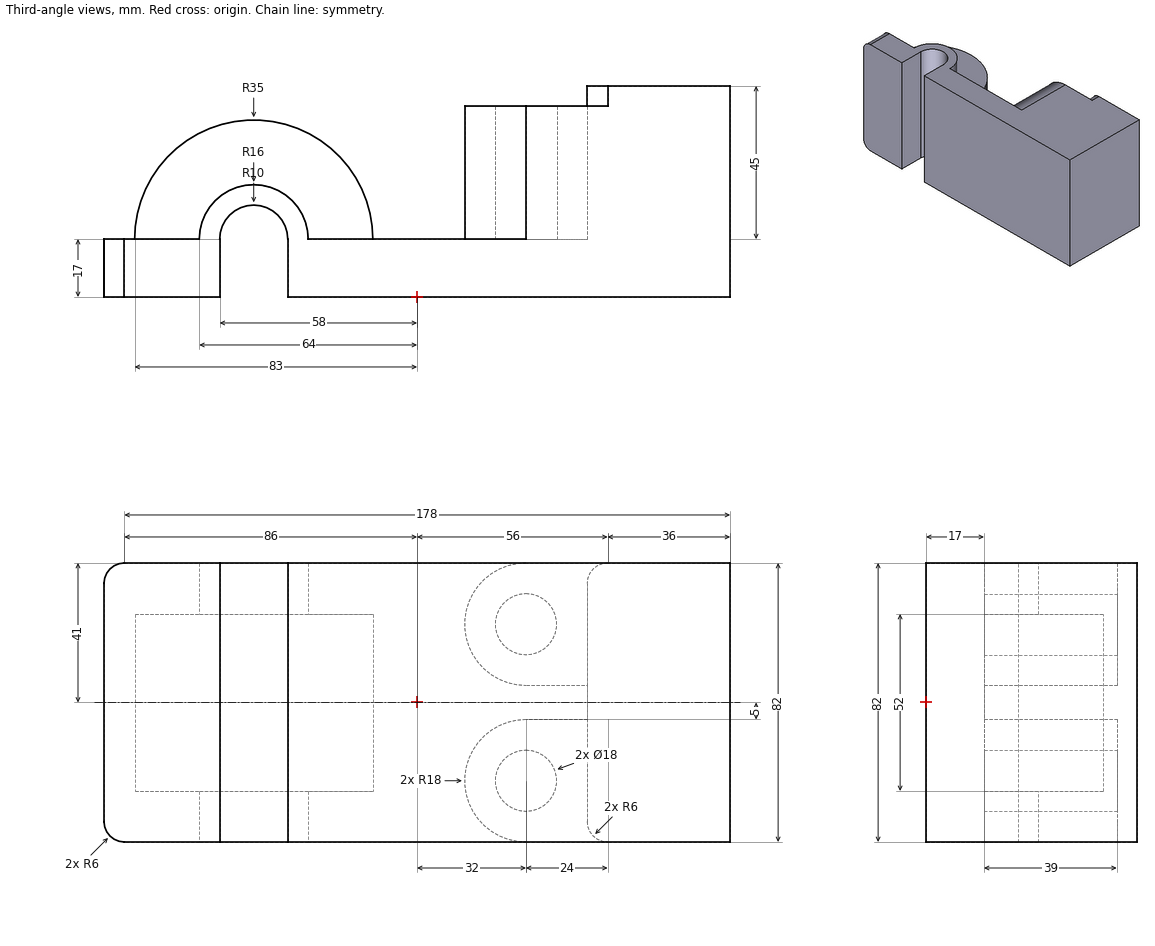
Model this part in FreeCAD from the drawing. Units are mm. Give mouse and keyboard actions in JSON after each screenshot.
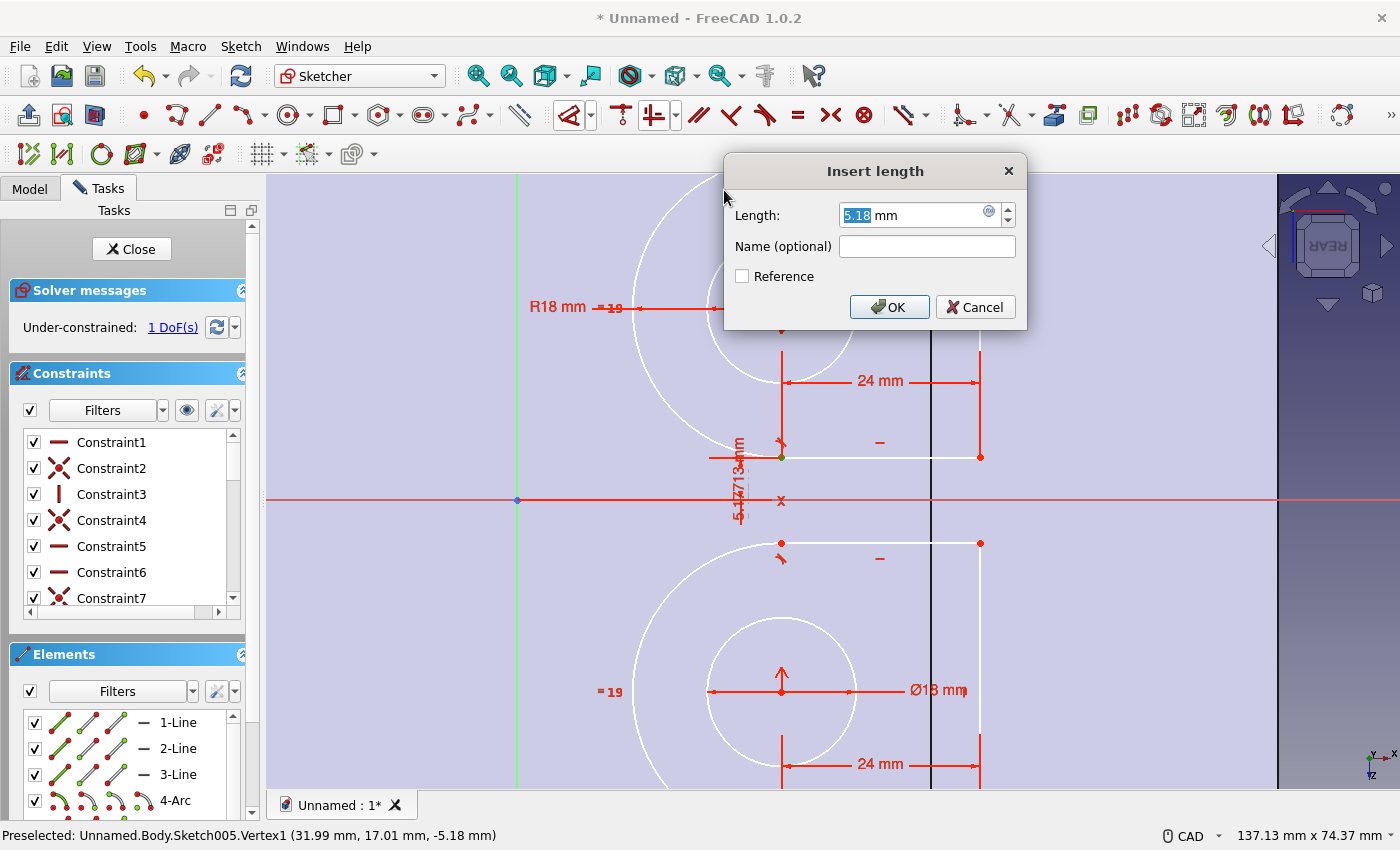
{"action": "type", "text": "5"}
{"action": "key", "text": "Return"}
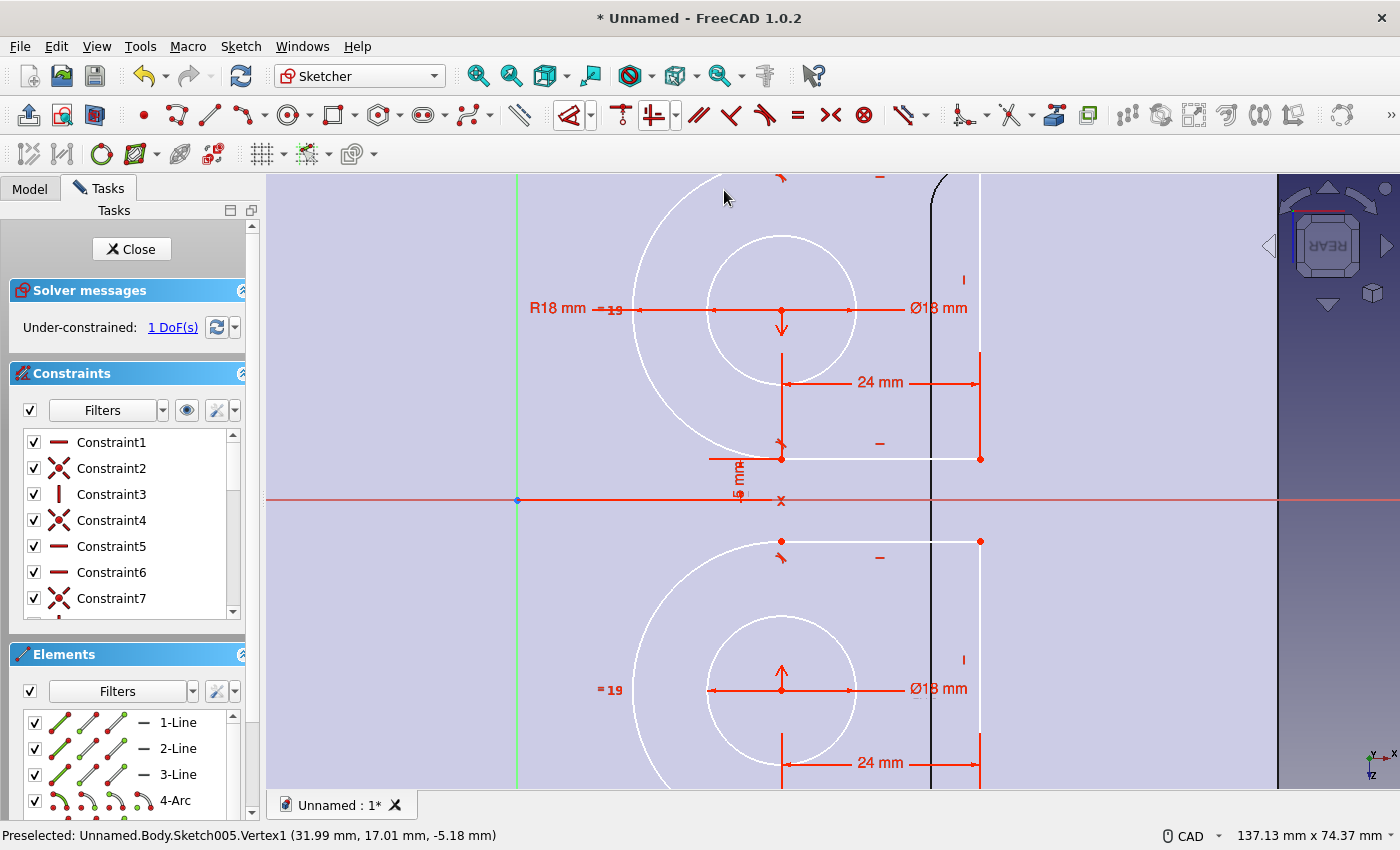
{"action": "left_click", "coordinate": [782, 310]}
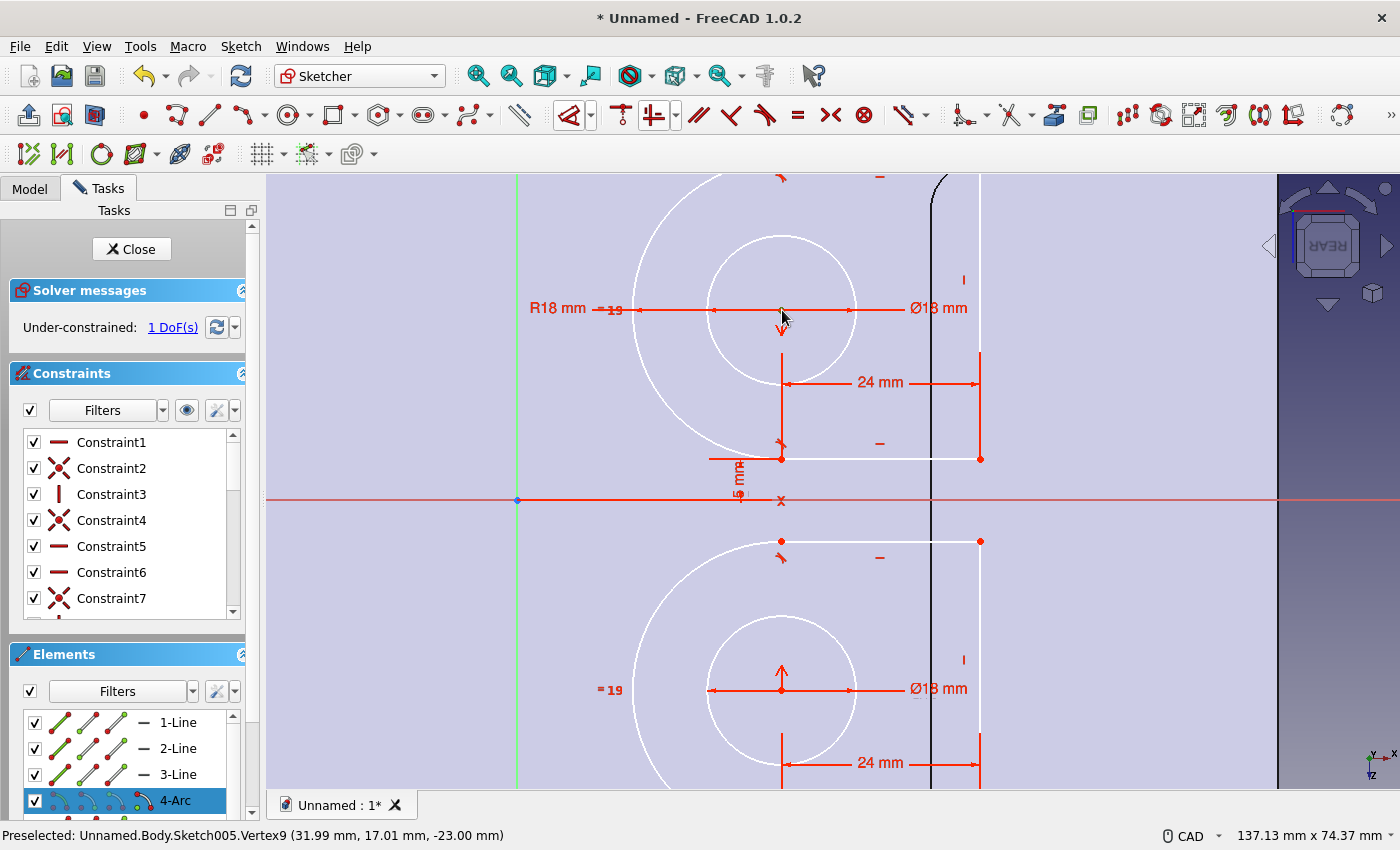
{"action": "left_click", "coordinate": [590, 116]}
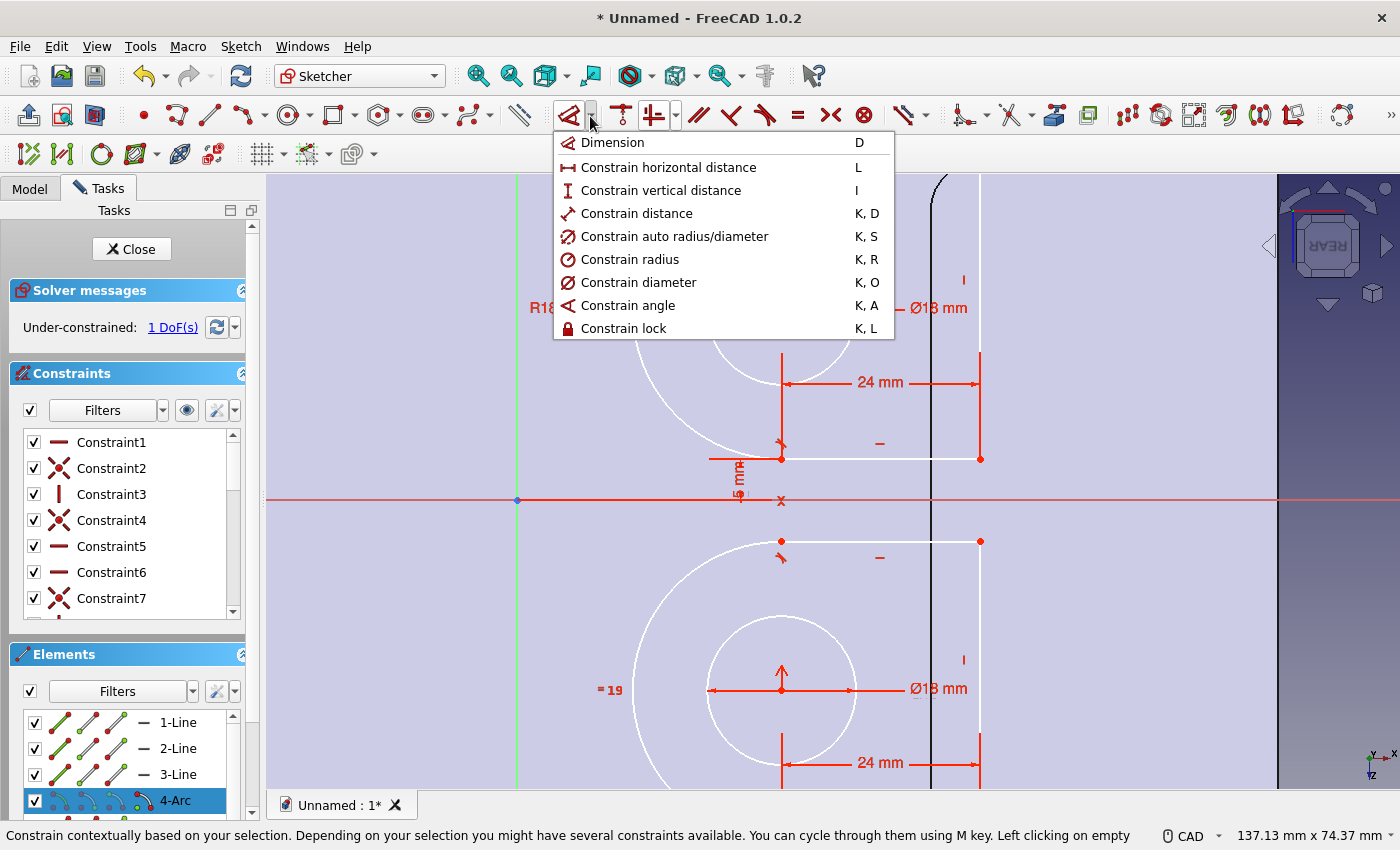
{"action": "left_click", "coordinate": [724, 168]}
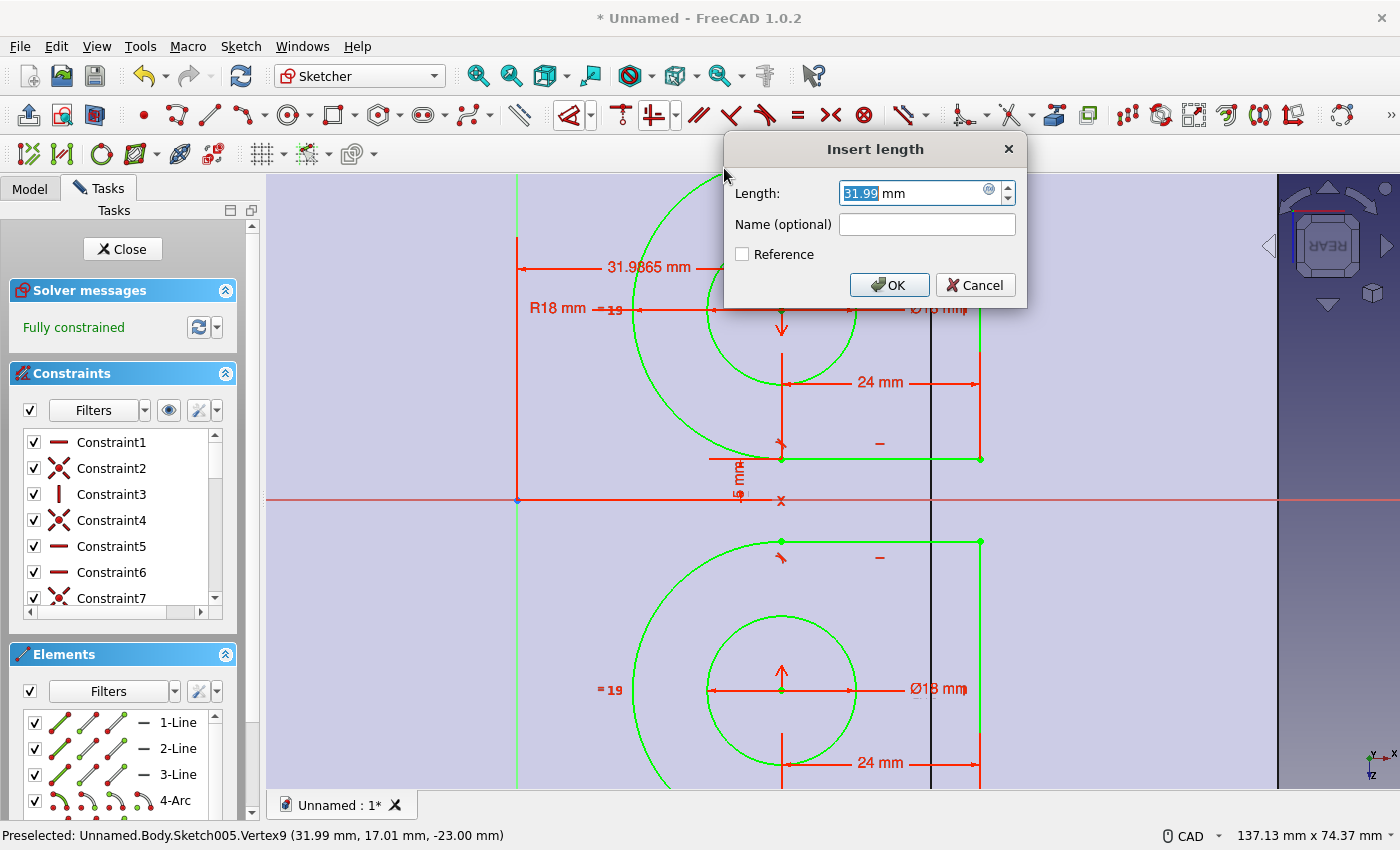
{"action": "type", "text": "32"}
{"action": "key", "text": "Return"}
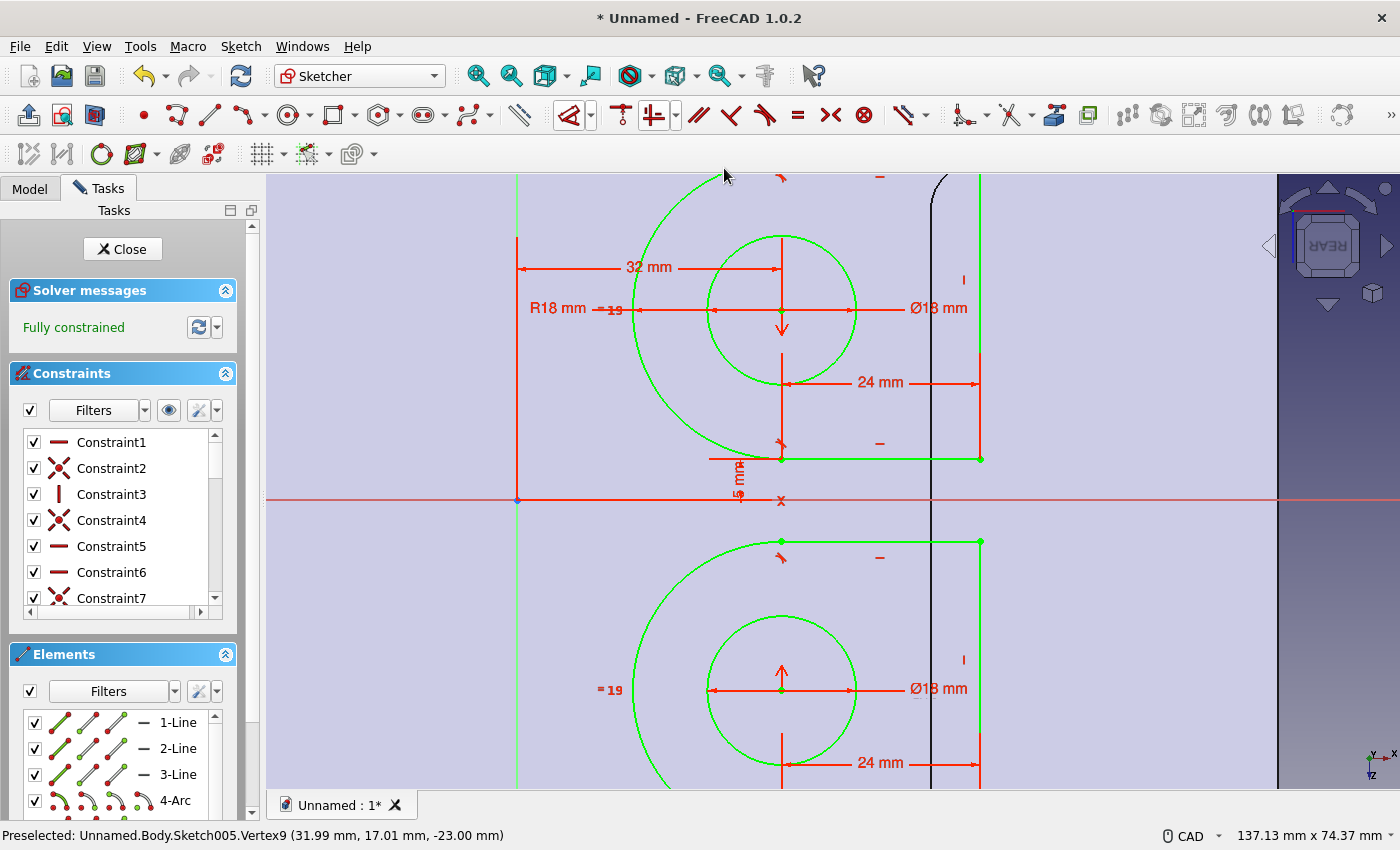
{"action": "left_click", "coordinate": [123, 249]}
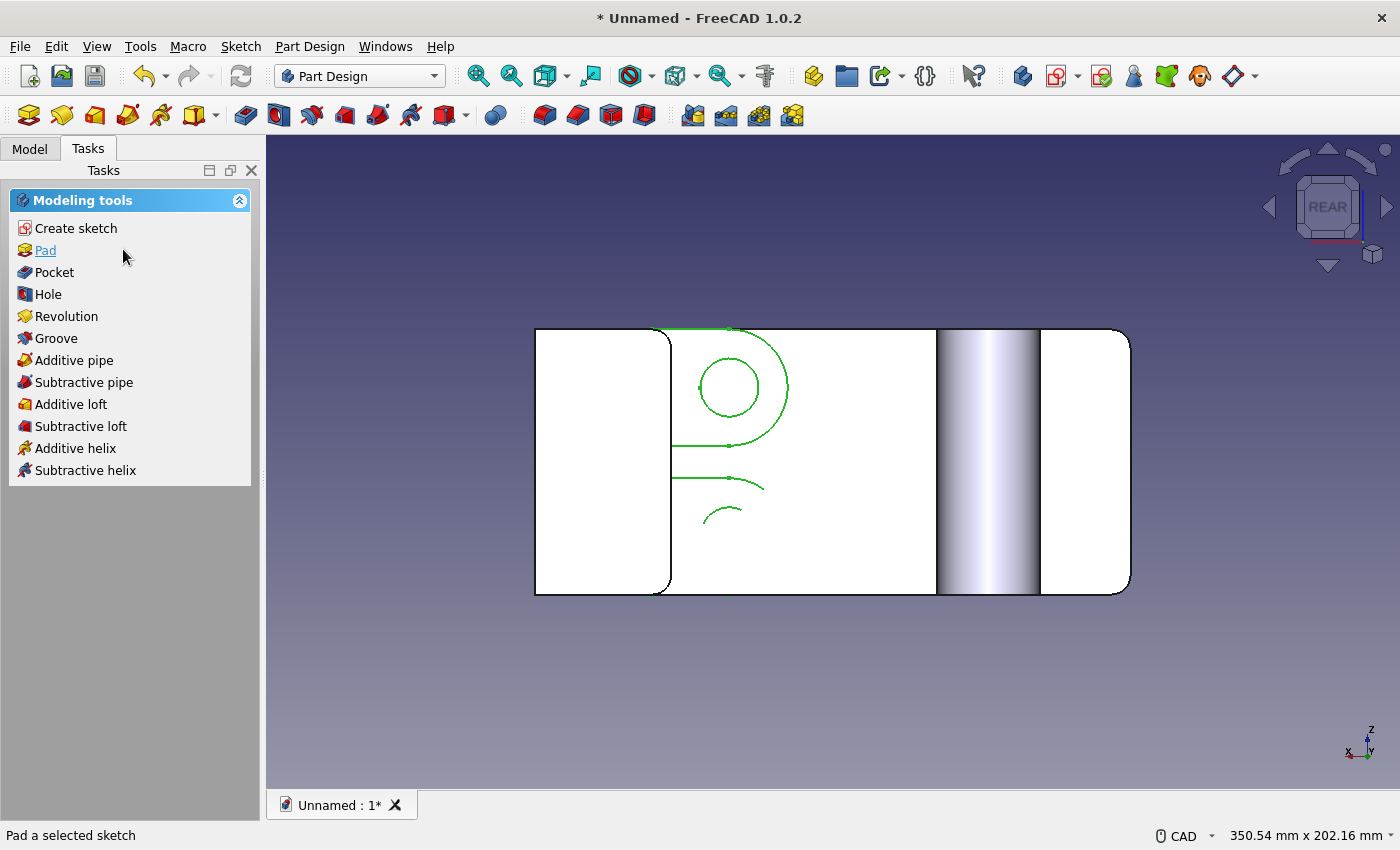
{"action": "left_click", "coordinate": [29, 116]}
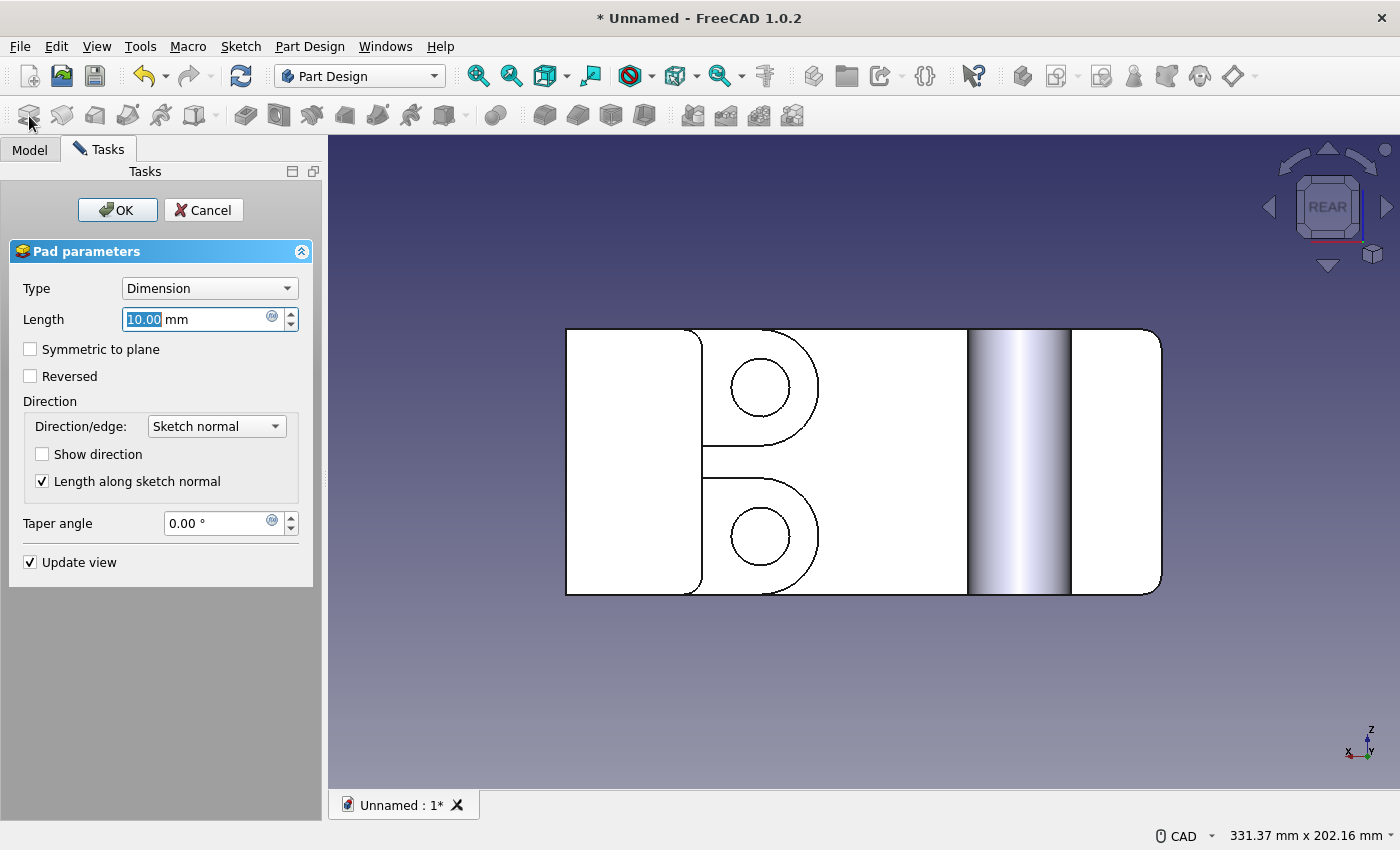
{"action": "type", "text": "39"}
{"action": "key", "text": "Tab"}